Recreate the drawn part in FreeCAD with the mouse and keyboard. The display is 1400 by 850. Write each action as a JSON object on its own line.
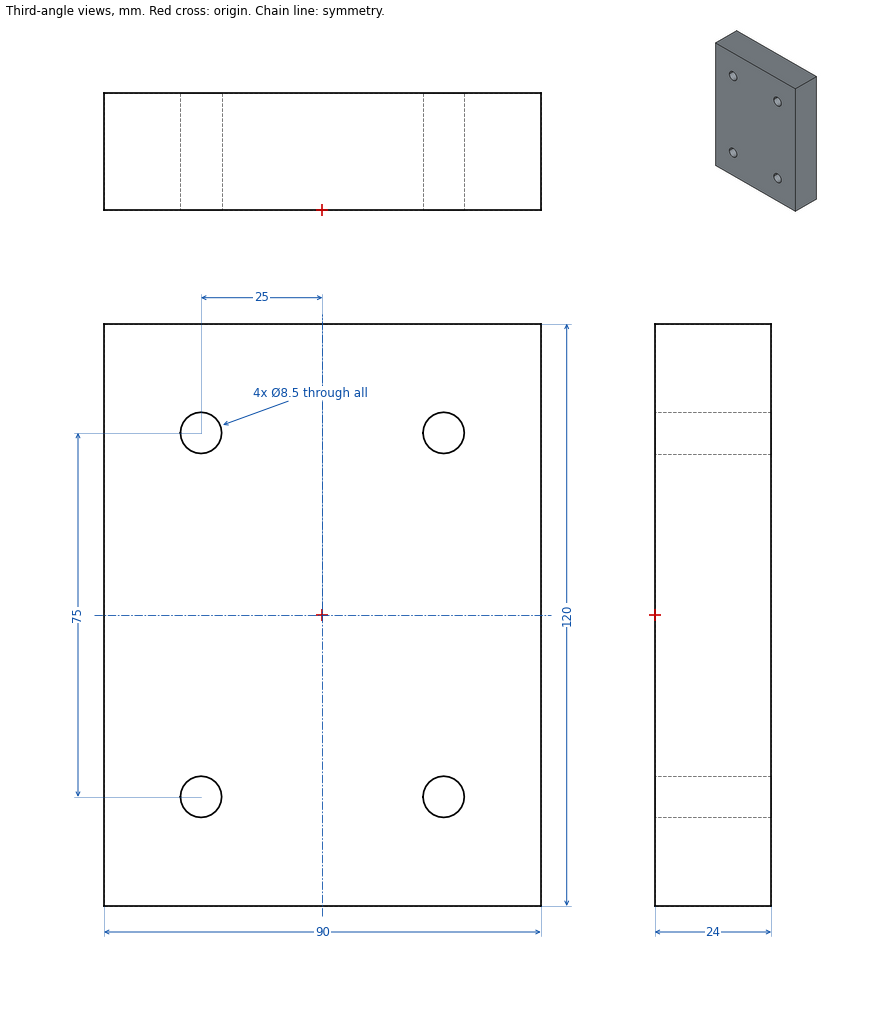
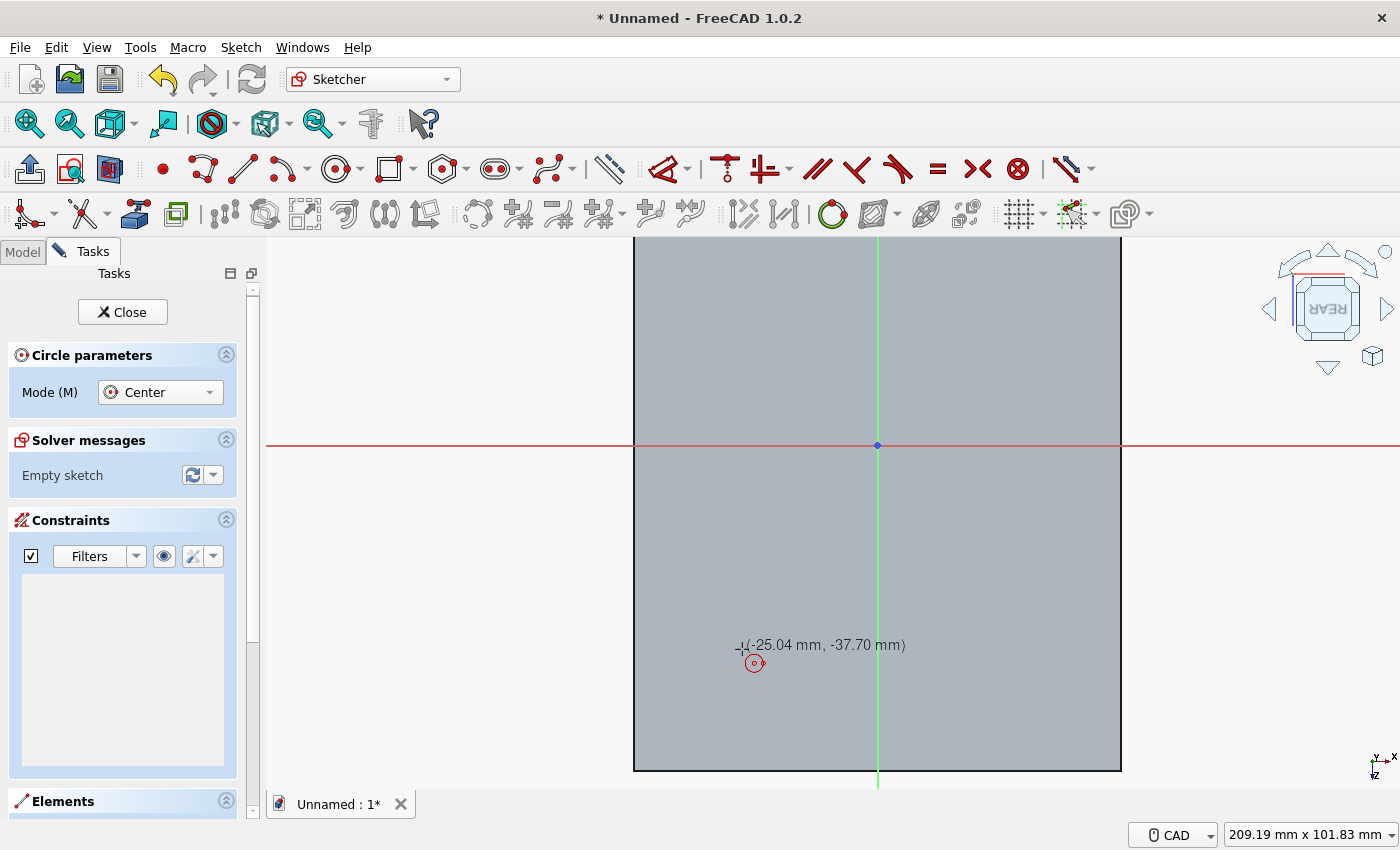
{"action": "left_click", "coordinate": [742, 649]}
{"action": "left_click", "coordinate": [758, 633]}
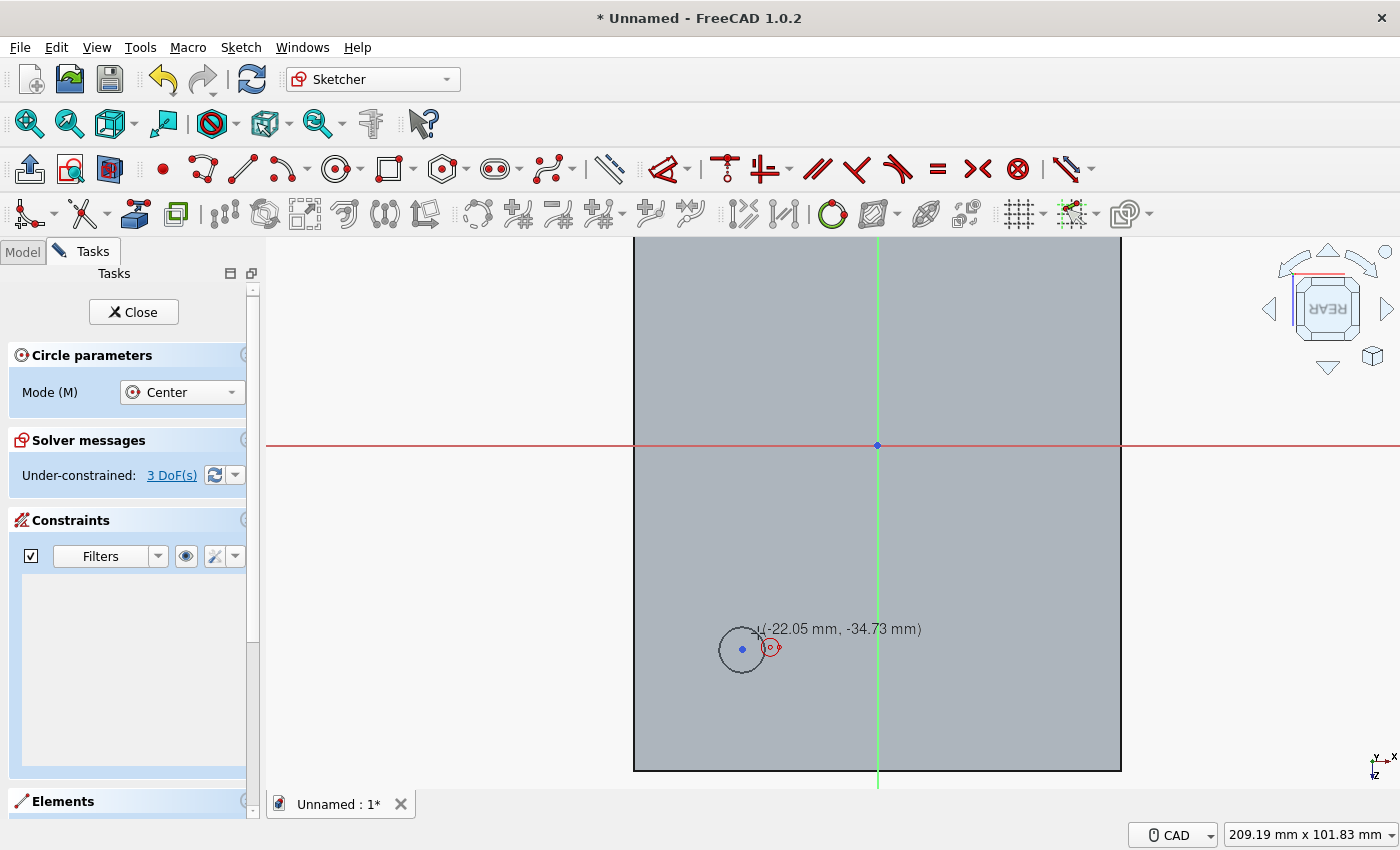
{"action": "scroll", "coordinate": [294, 761], "scroll_direction": "down", "scroll_amount": 1}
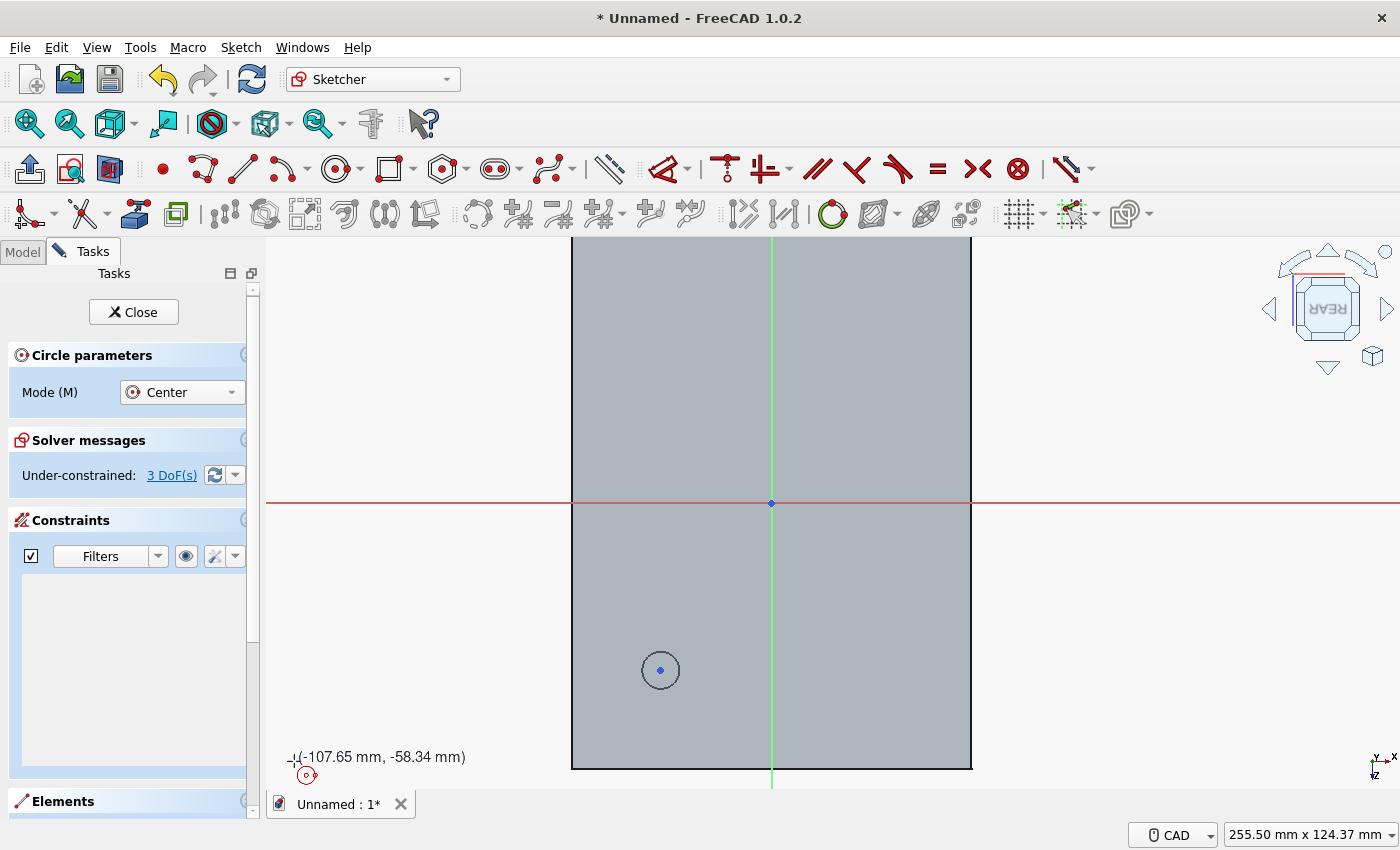
{"action": "left_click", "coordinate": [661, 337]}
{"action": "left_click", "coordinate": [674, 323]}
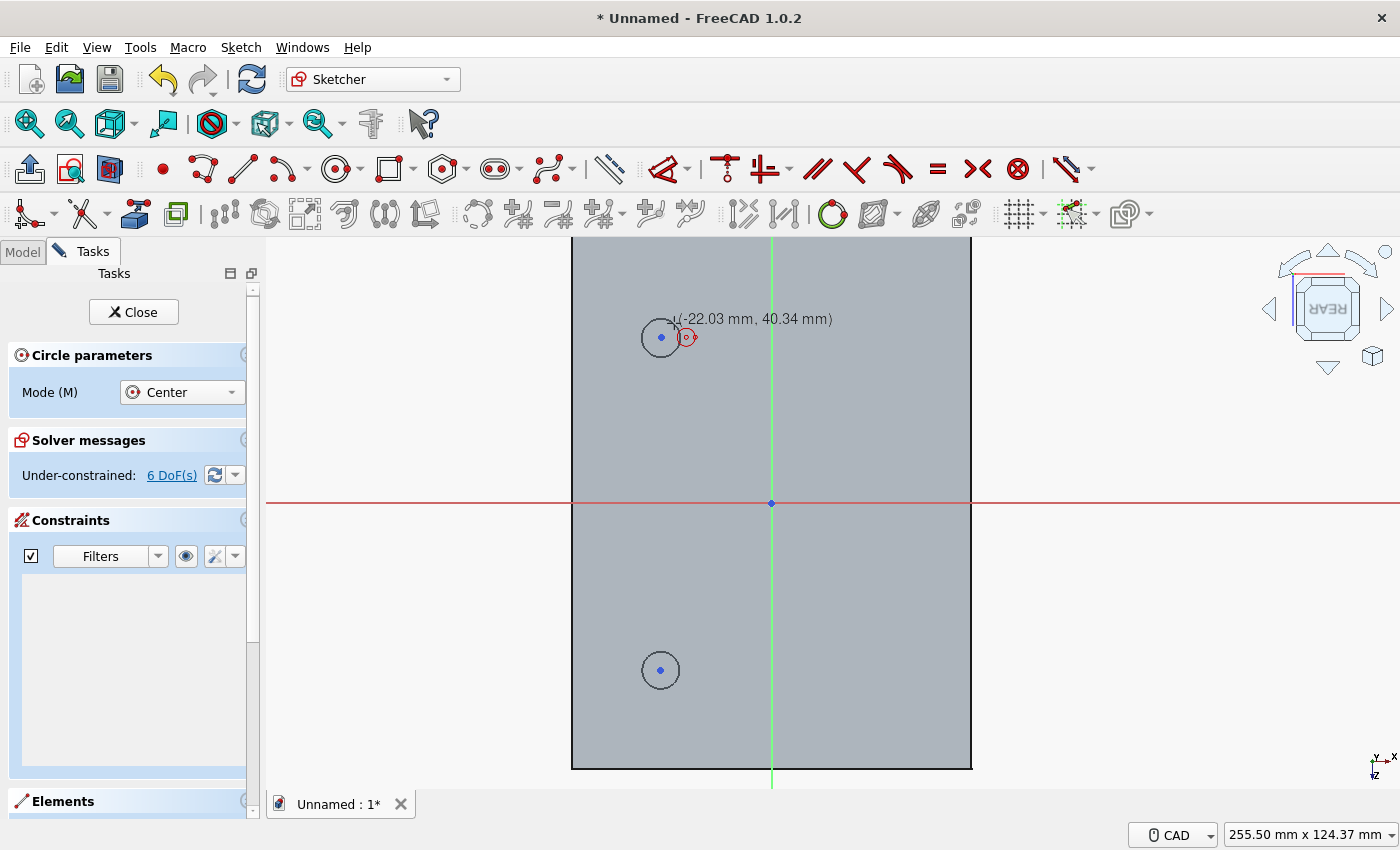
{"action": "left_click", "coordinate": [883, 337]}
{"action": "left_click", "coordinate": [896, 323]}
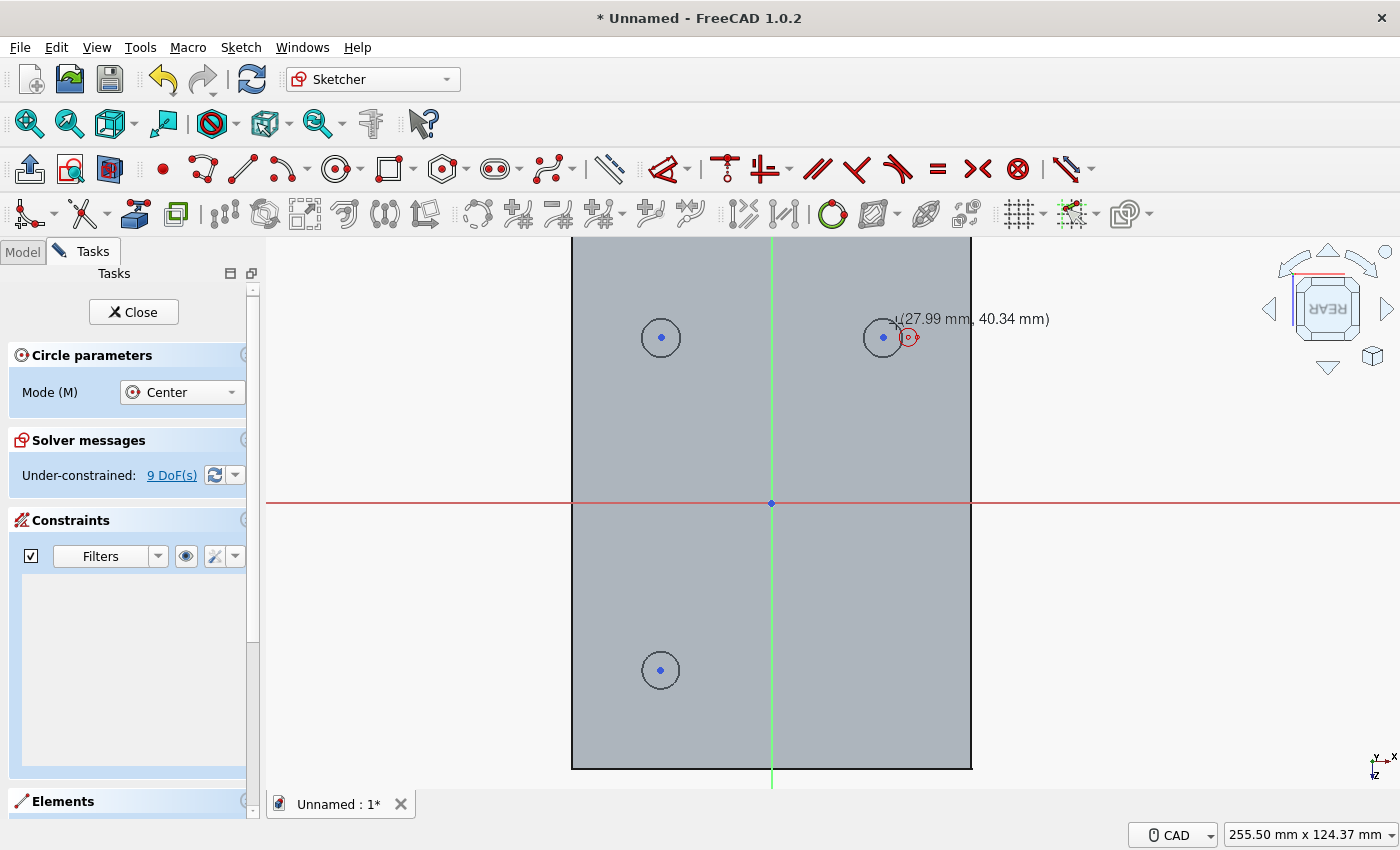
{"action": "left_click", "coordinate": [883, 669]}
{"action": "left_click", "coordinate": [896, 656]}
{"action": "key", "text": "Escape"}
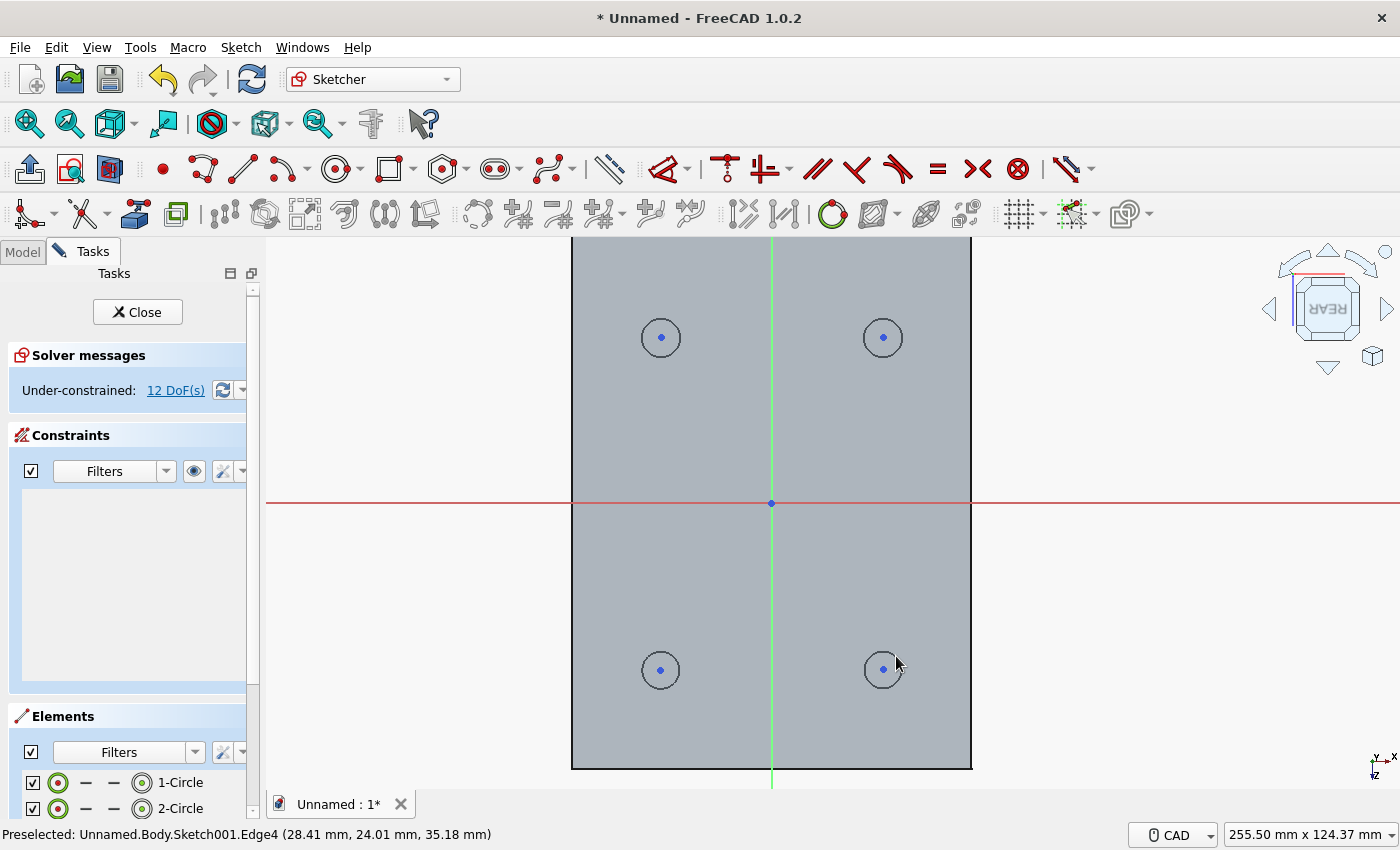
{"action": "left_click", "coordinate": [674, 657]}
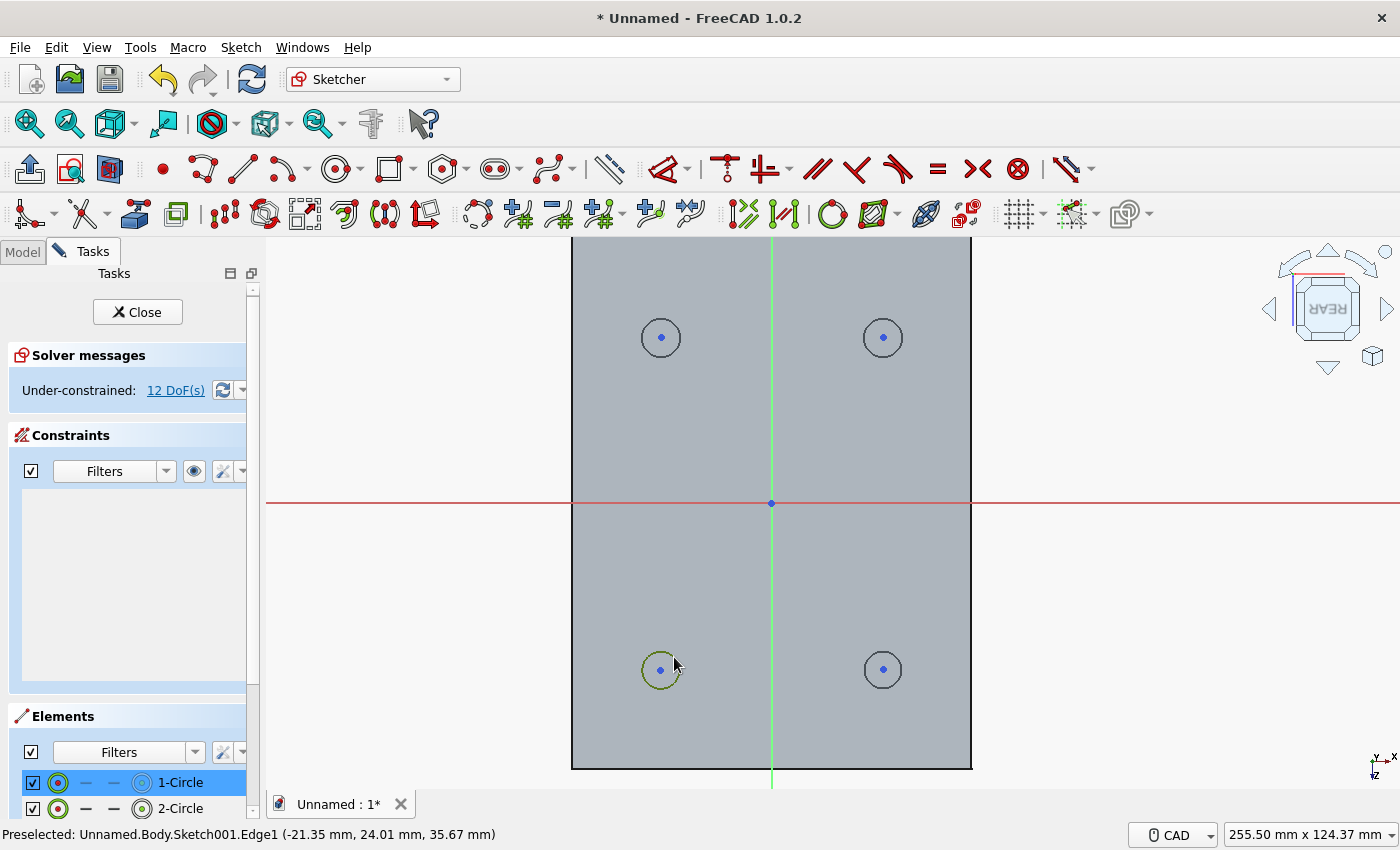
{"action": "left_click", "coordinate": [674, 324]}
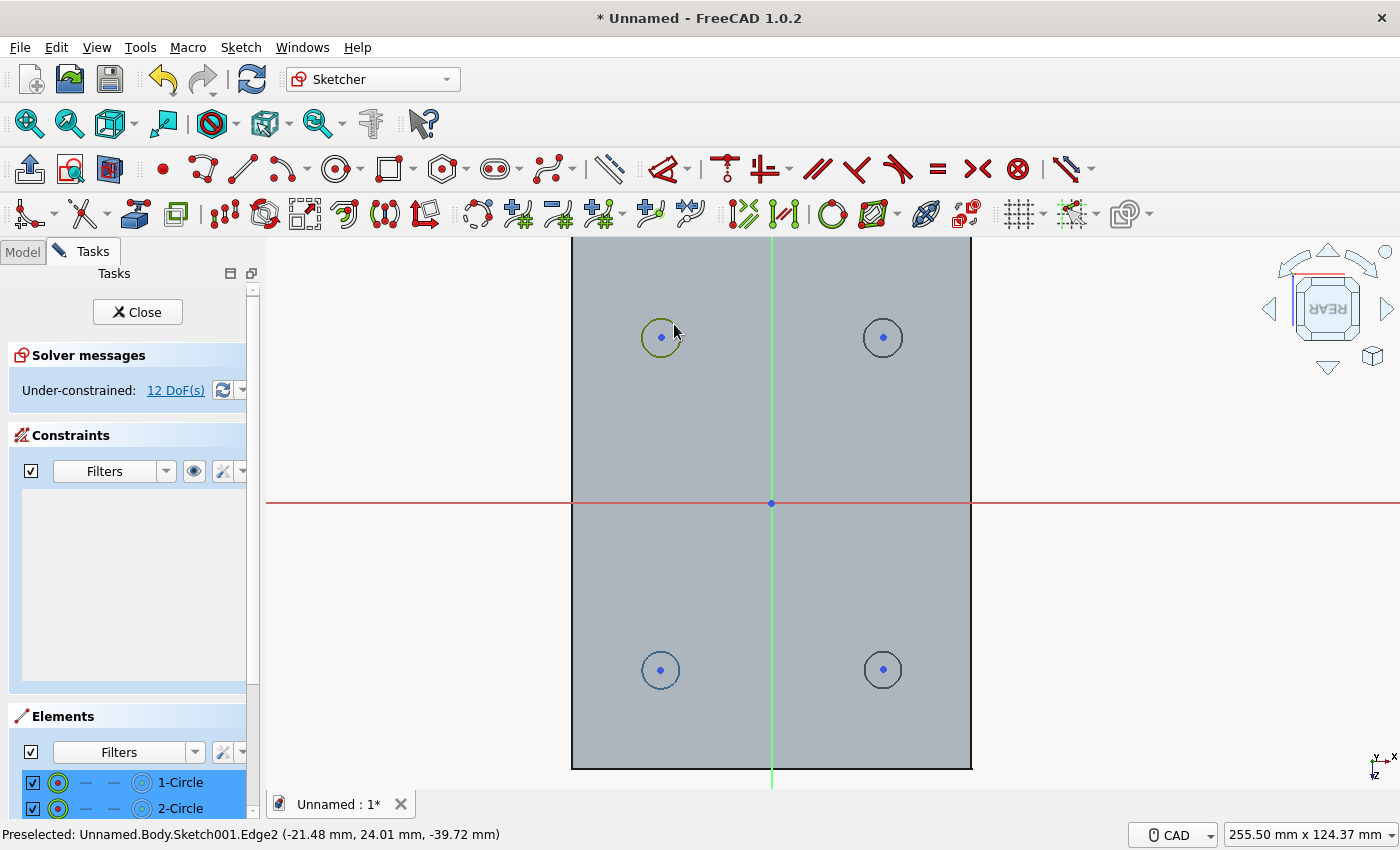
{"action": "left_click", "coordinate": [896, 324]}